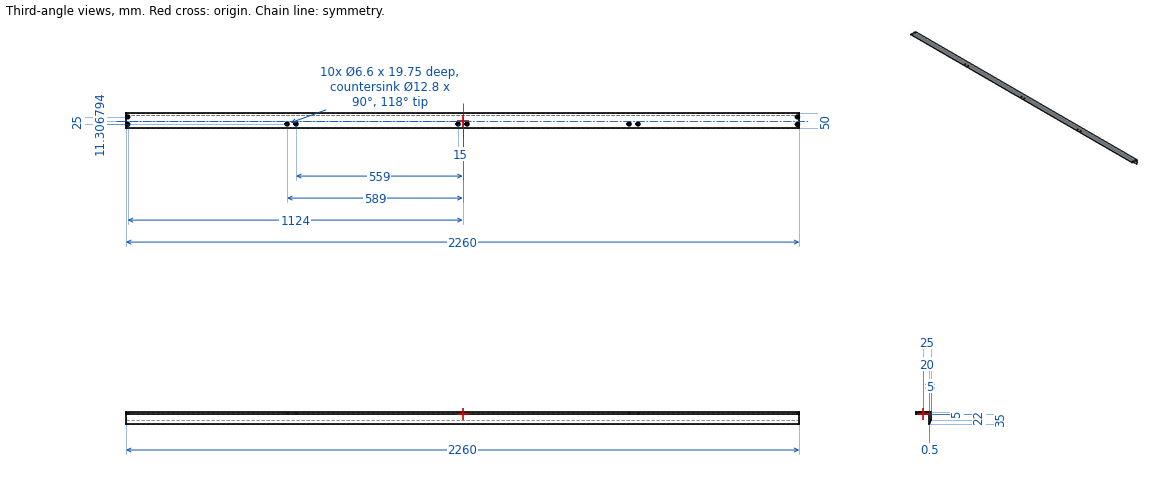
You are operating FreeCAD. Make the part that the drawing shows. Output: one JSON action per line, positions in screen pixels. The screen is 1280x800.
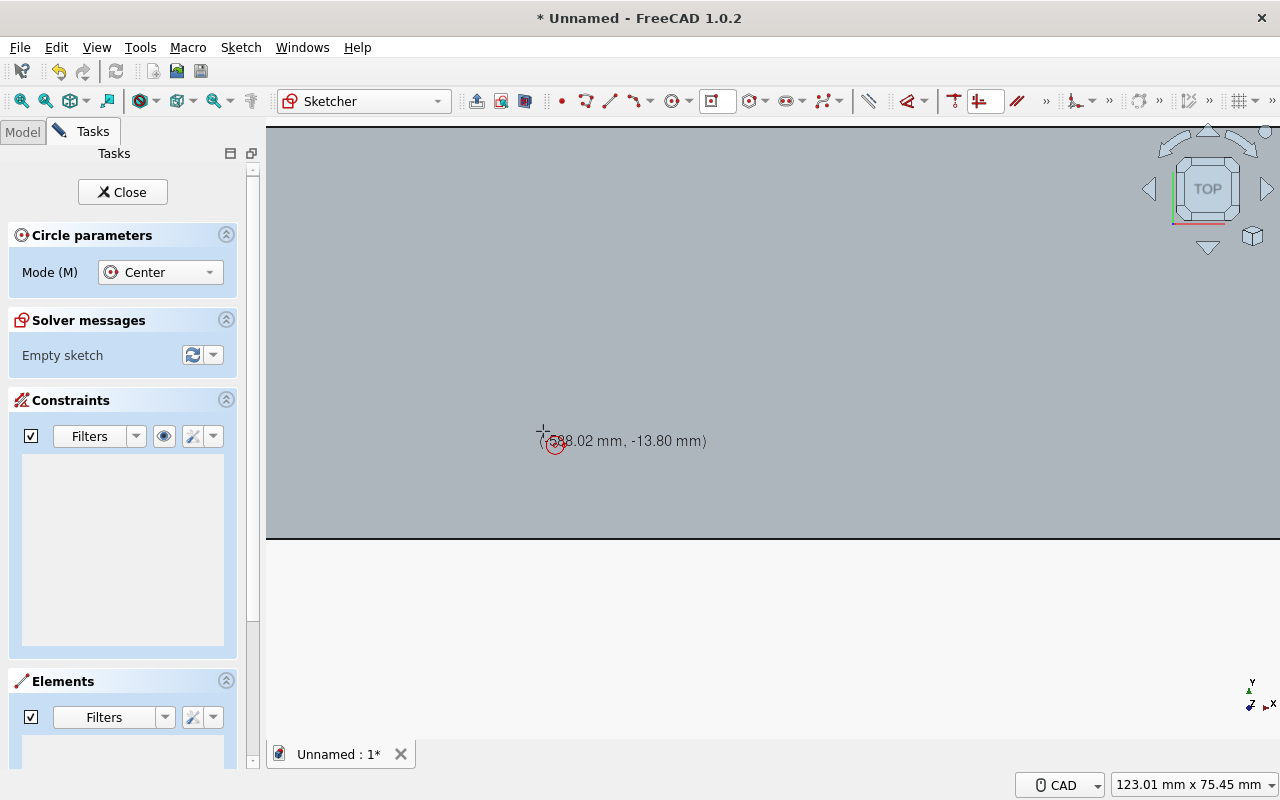
{"action": "scroll", "coordinate": [506, 432], "scroll_direction": "down", "scroll_amount": 16}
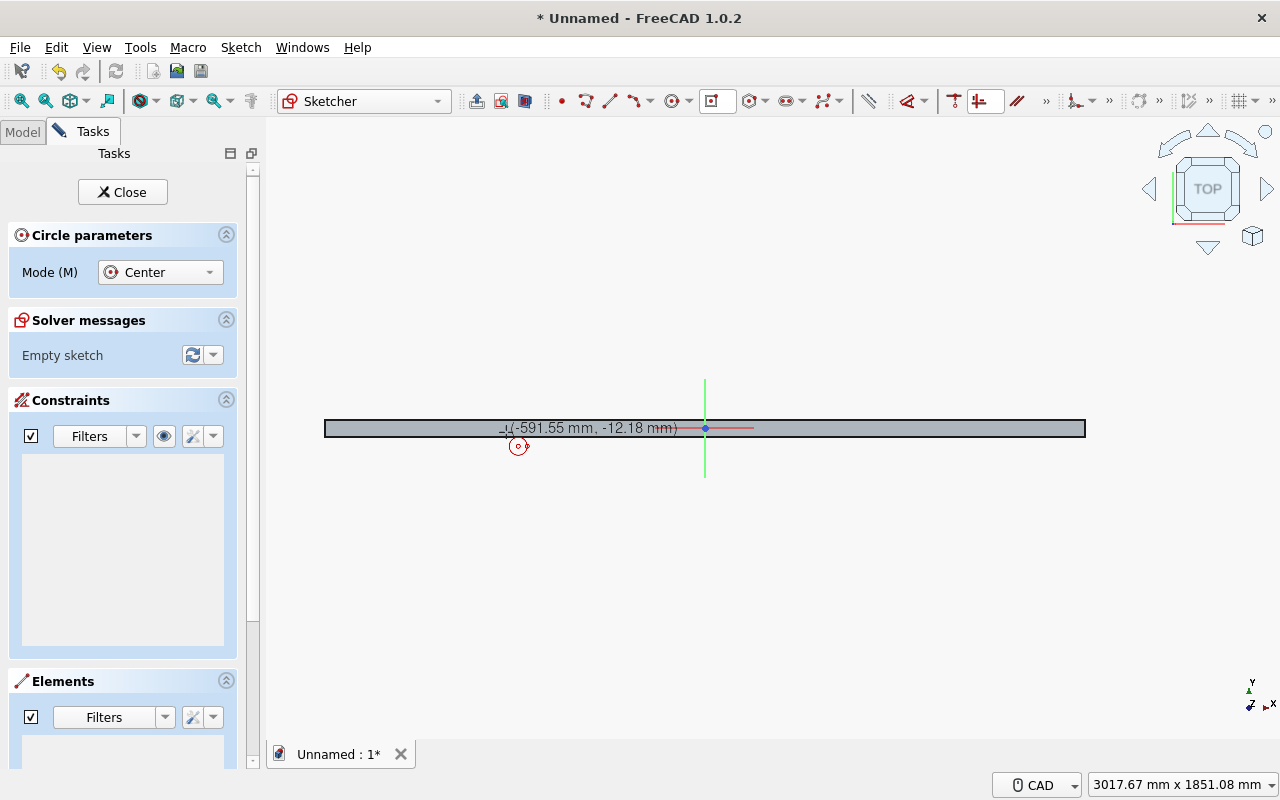
{"action": "scroll", "coordinate": [507, 432], "scroll_direction": "up", "scroll_amount": 8}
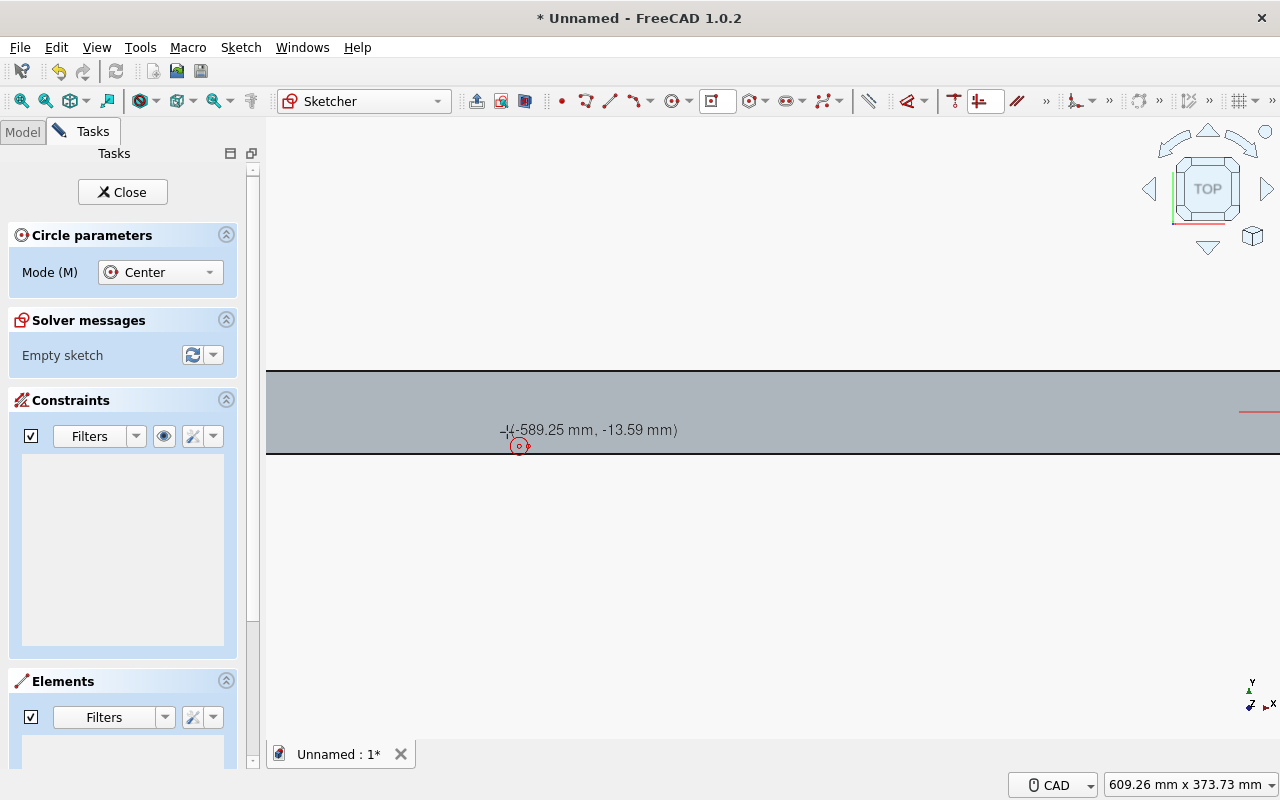
{"action": "left_click", "coordinate": [506, 431]}
{"action": "mouse_move", "coordinate": [510, 427]}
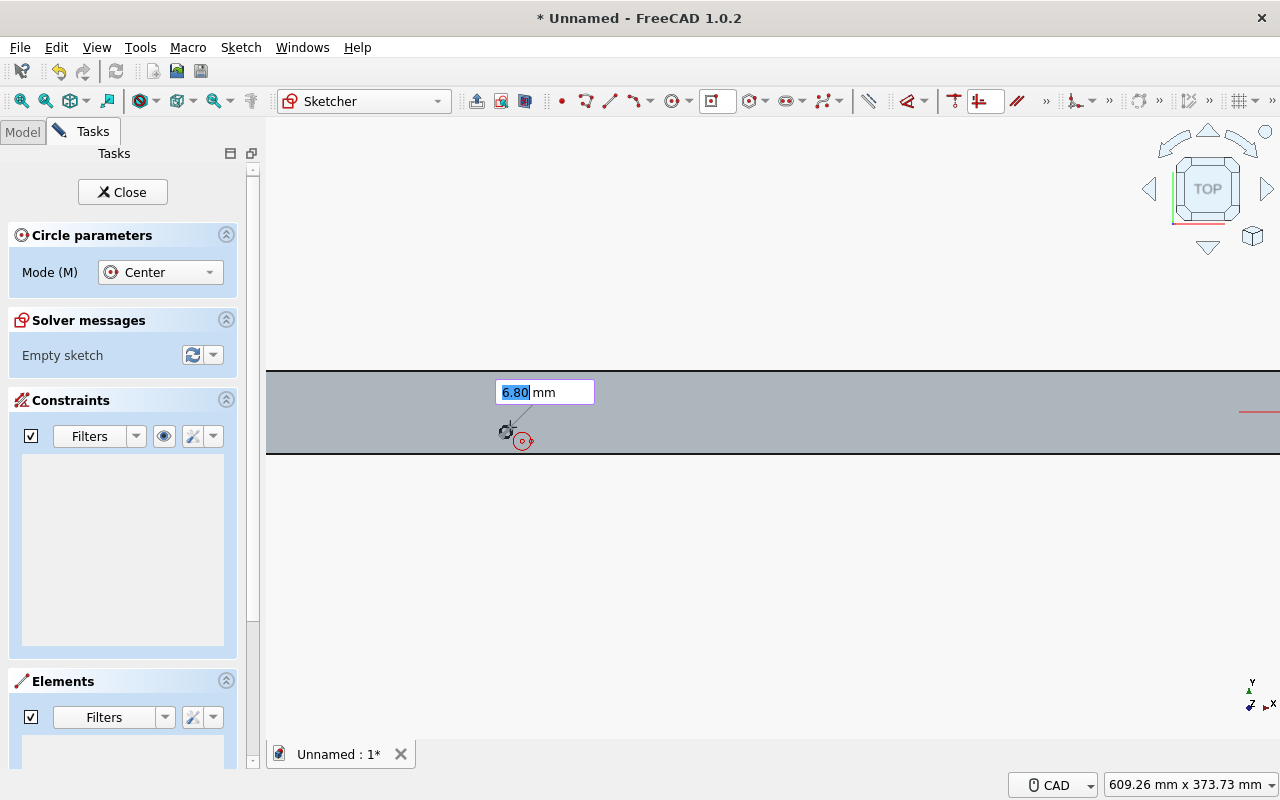
{"action": "type", "text": "6.6"}
{"action": "key", "text": "Return"}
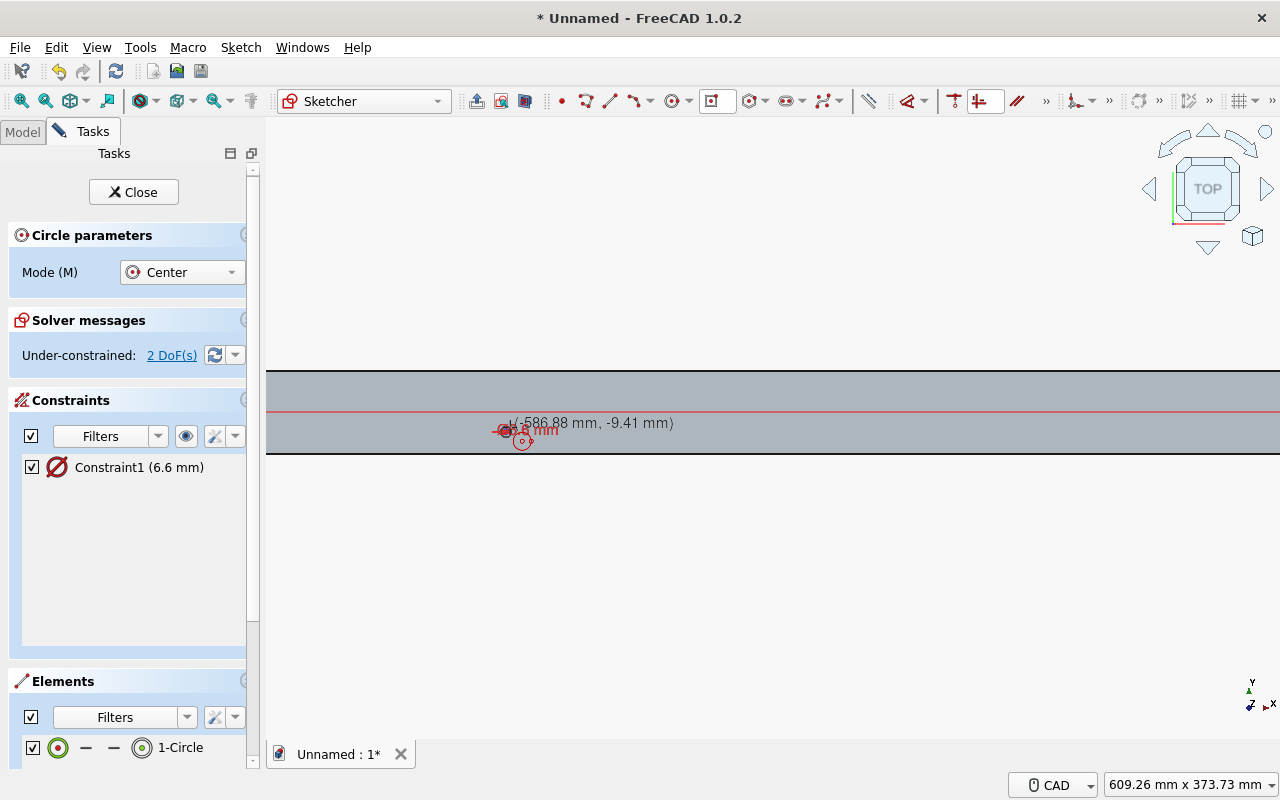
{"action": "scroll", "coordinate": [556, 431], "scroll_direction": "up", "scroll_amount": 8}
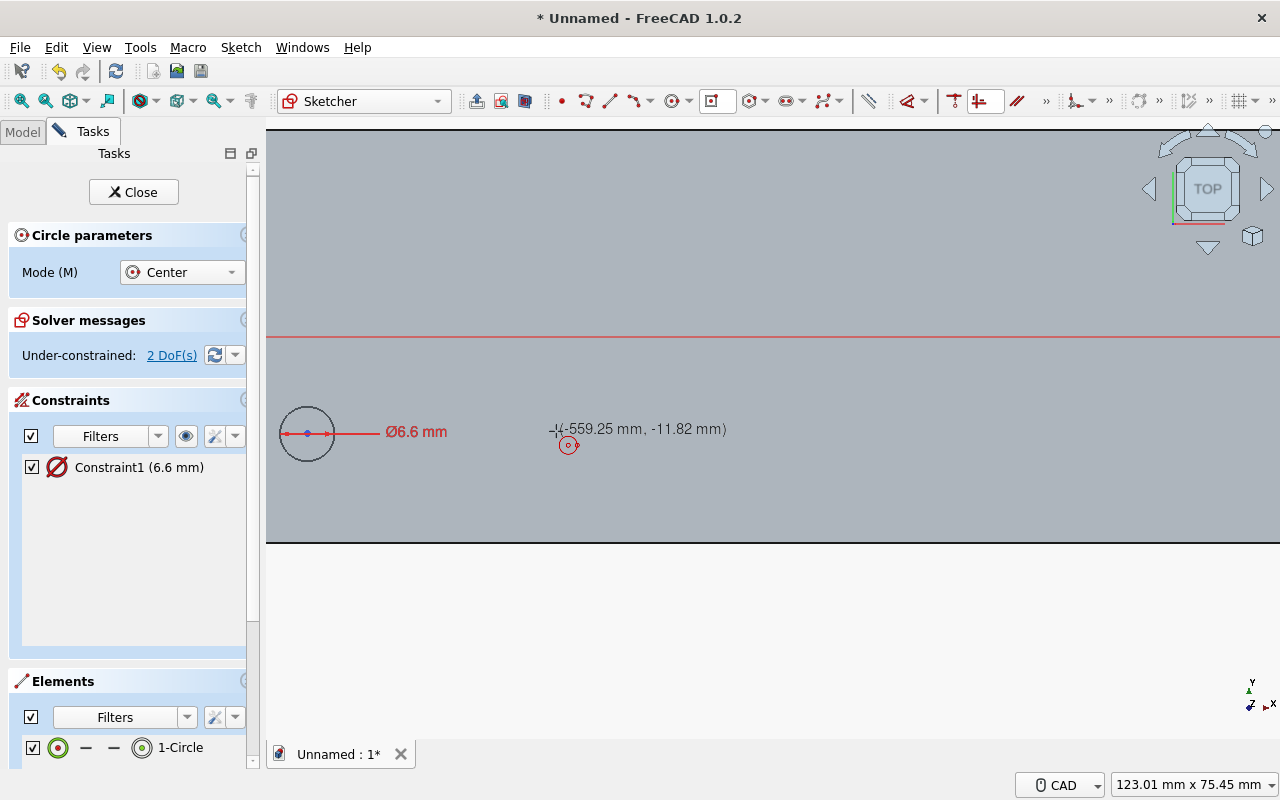
{"action": "scroll", "coordinate": [515, 432], "scroll_direction": "down", "scroll_amount": 16}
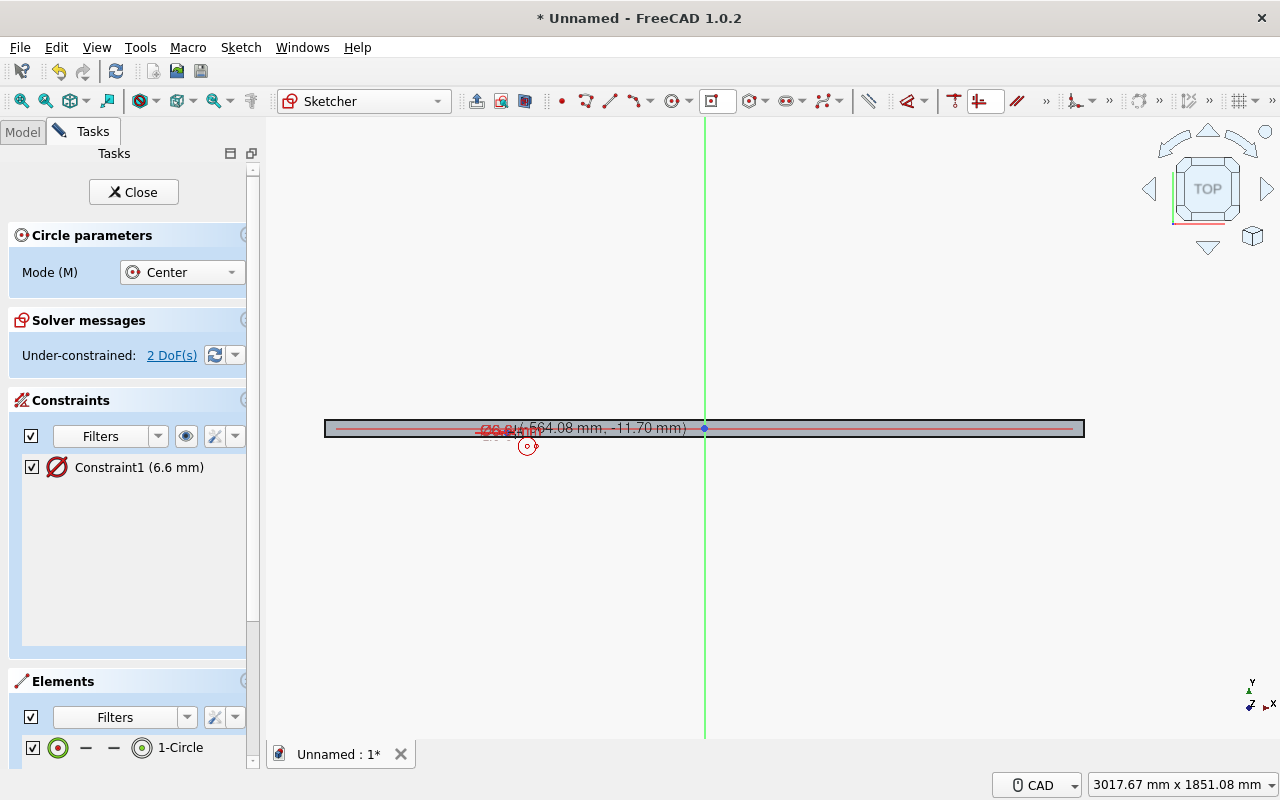
{"action": "scroll", "coordinate": [517, 432], "scroll_direction": "up", "scroll_amount": 8}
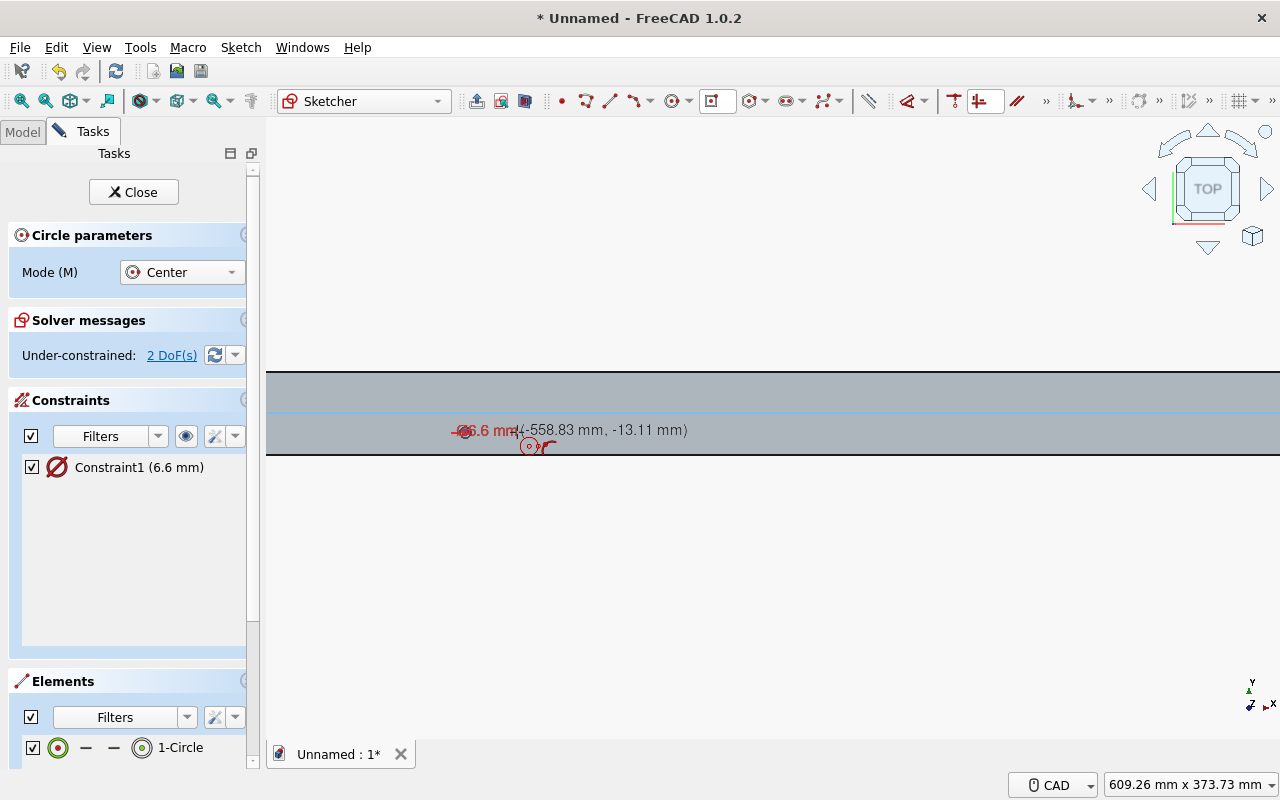
{"action": "left_click", "coordinate": [516, 432]}
{"action": "mouse_move", "coordinate": [520, 428]}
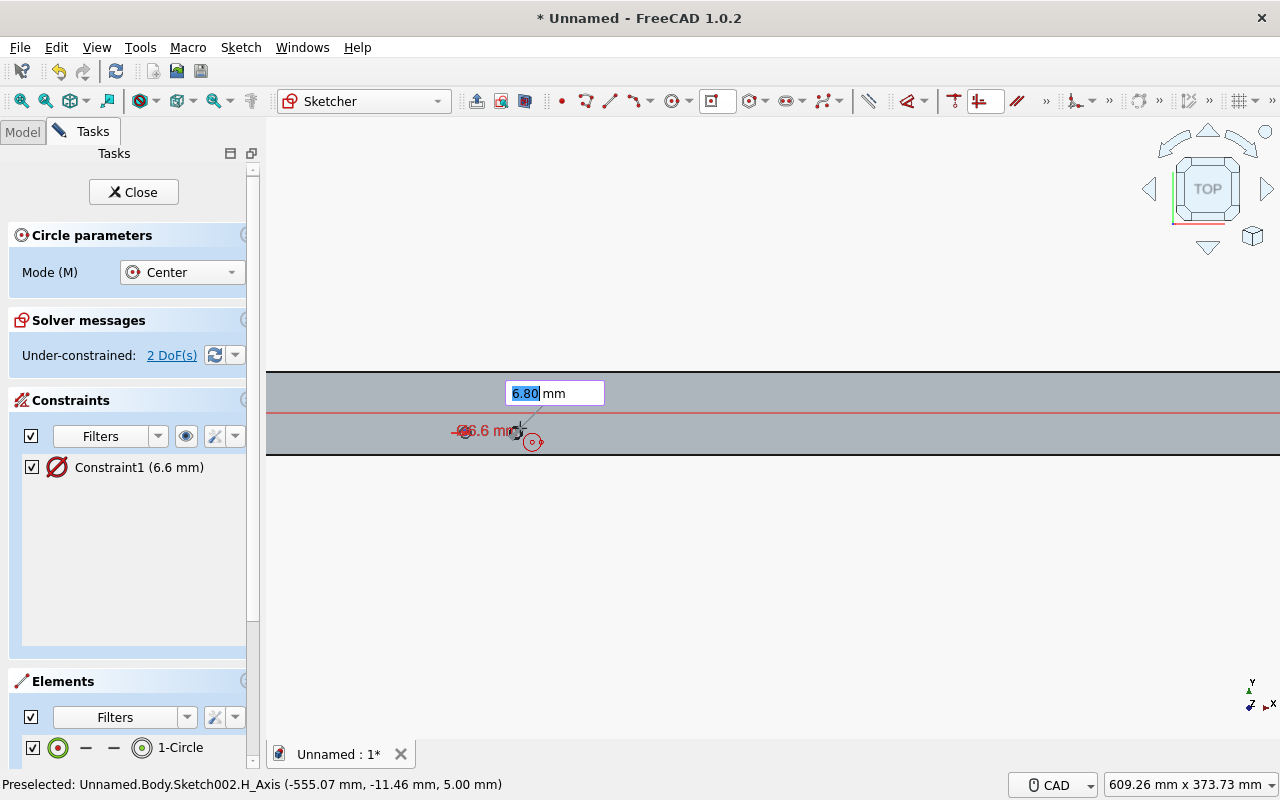
{"action": "type", "text": "6.6"}
{"action": "key", "text": "Return"}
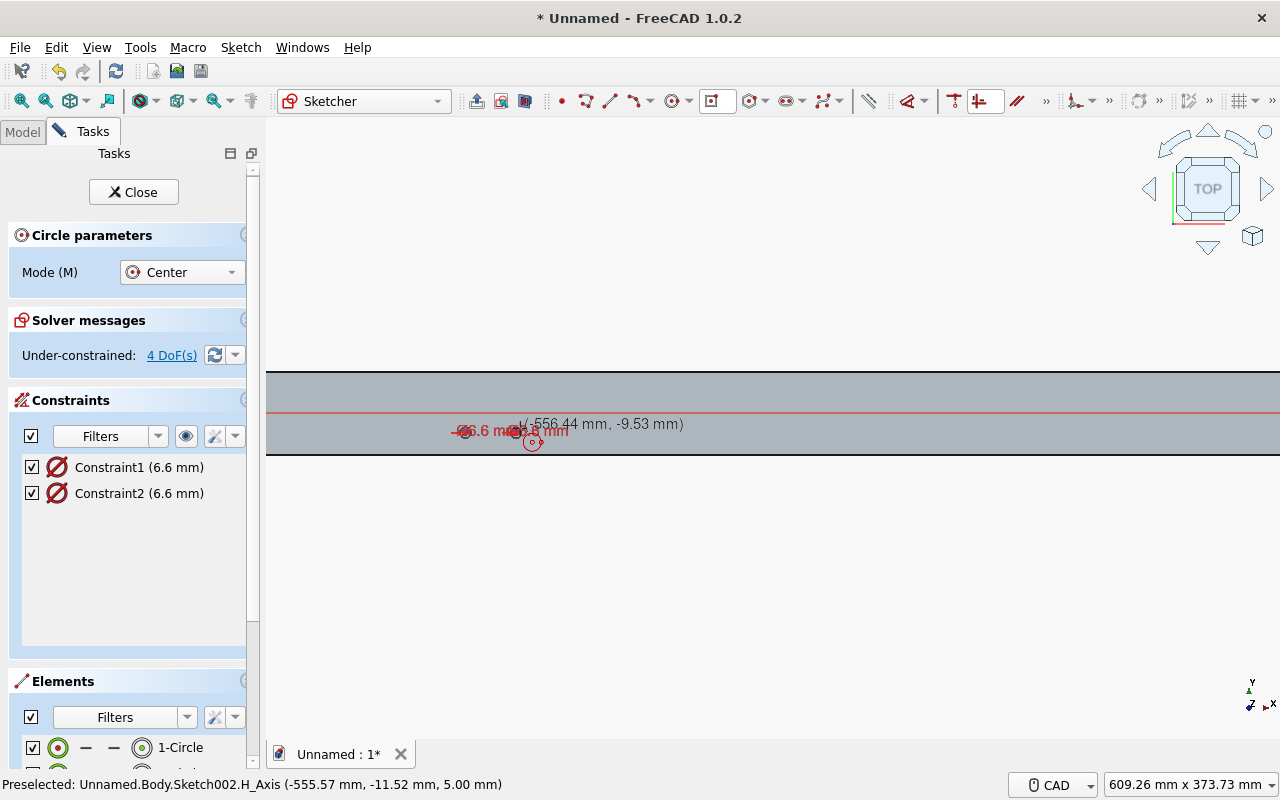
{"action": "scroll", "coordinate": [558, 431], "scroll_direction": "down", "scroll_amount": 9}